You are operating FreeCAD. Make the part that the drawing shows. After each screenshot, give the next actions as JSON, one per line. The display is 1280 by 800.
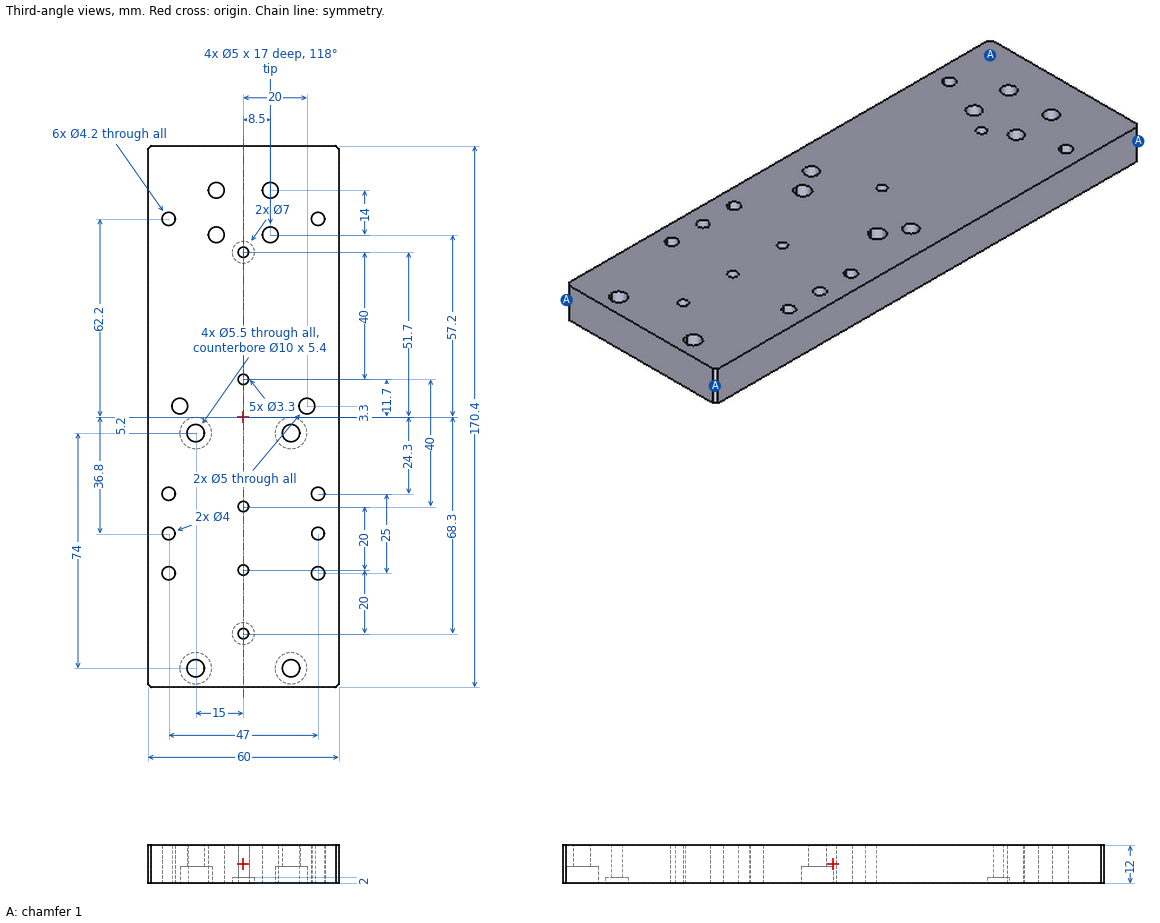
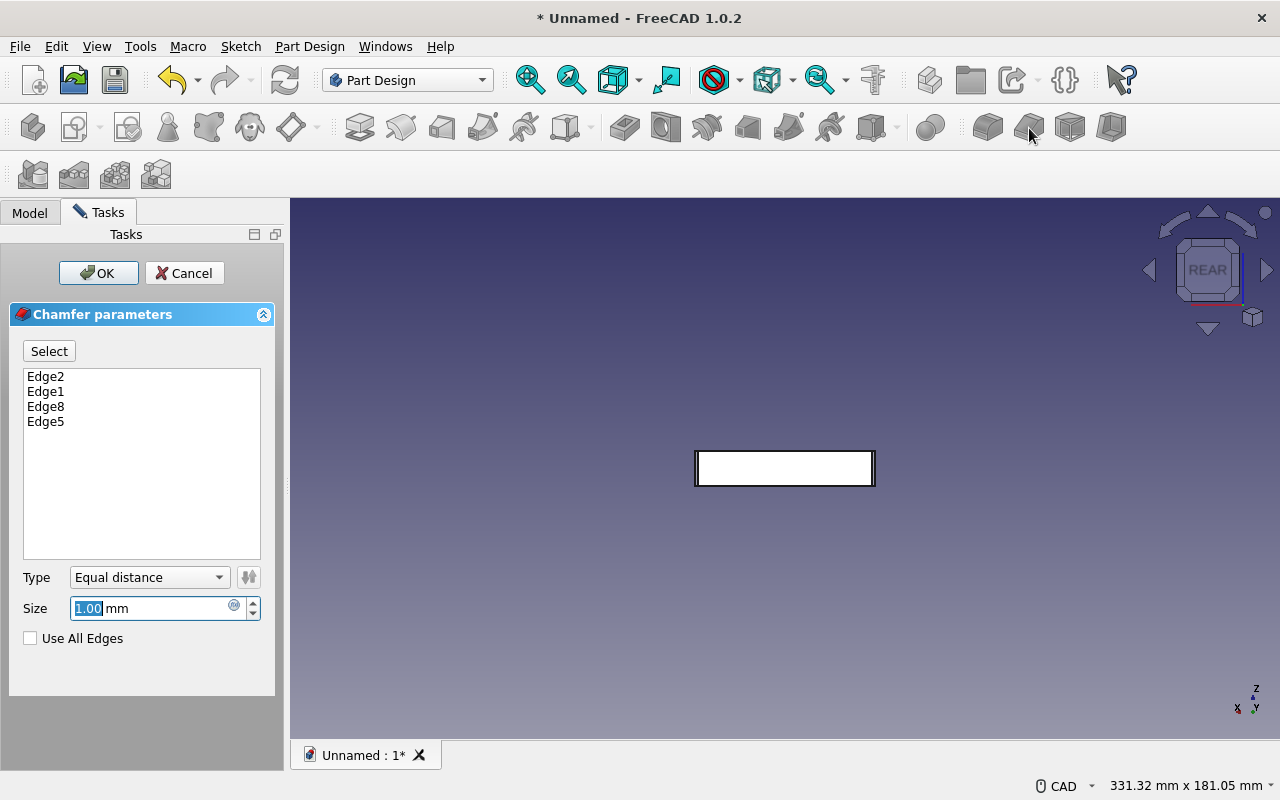
{"action": "type", "text": "1"}
{"action": "key", "text": "Tab"}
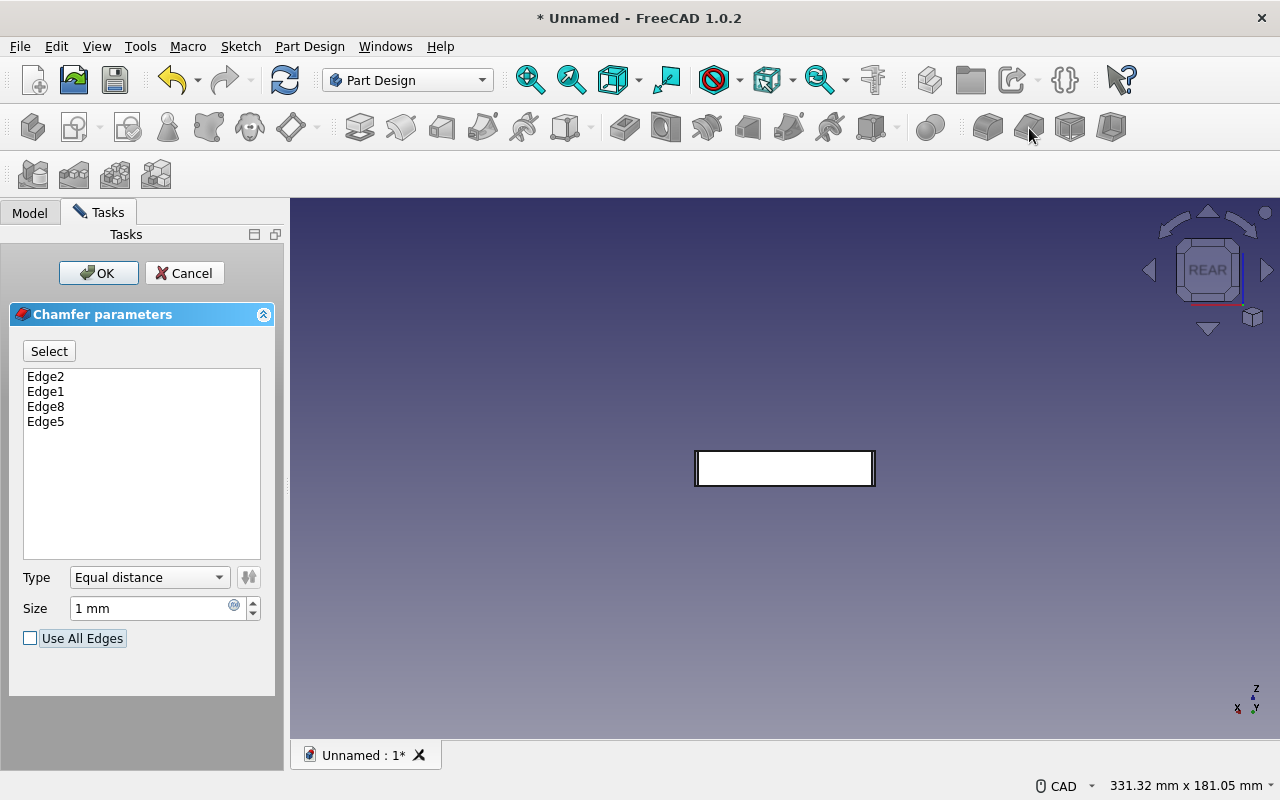
{"action": "left_click", "coordinate": [99, 273]}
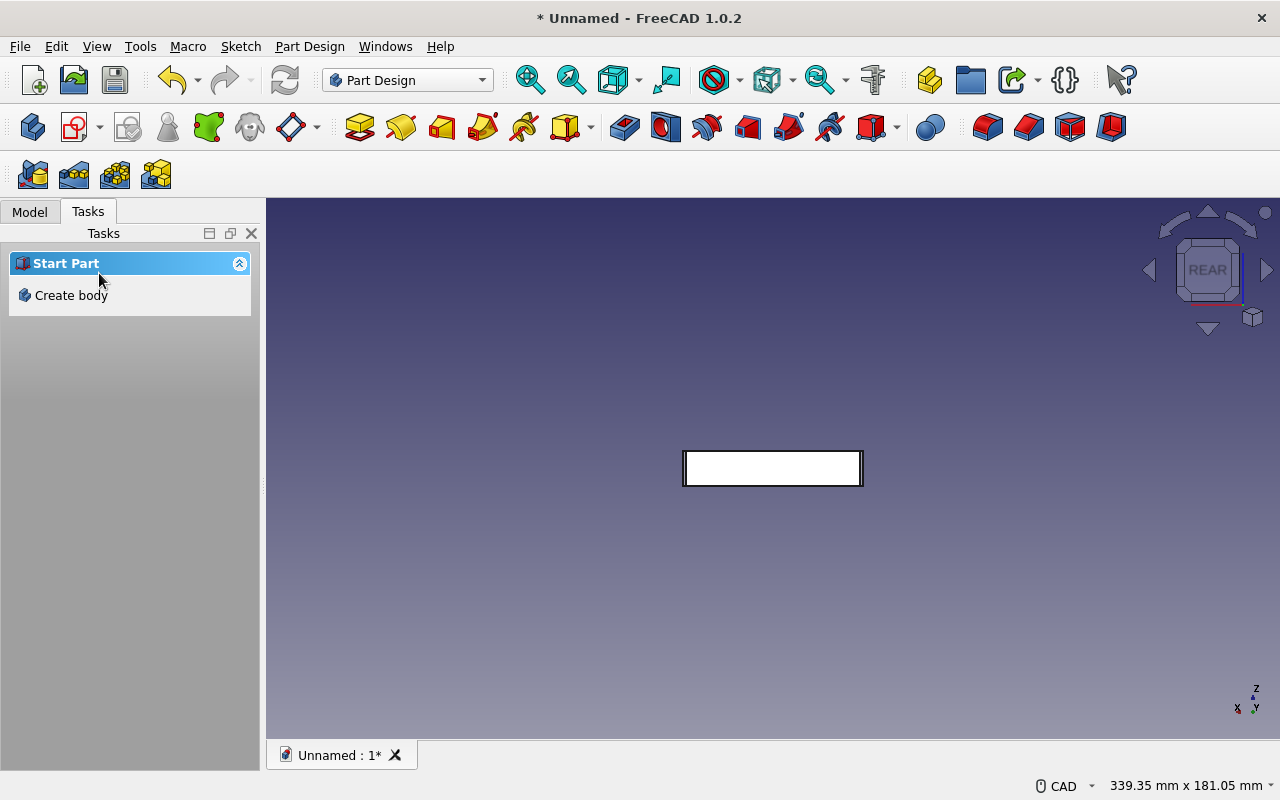
{"action": "left_click", "coordinate": [531, 80]}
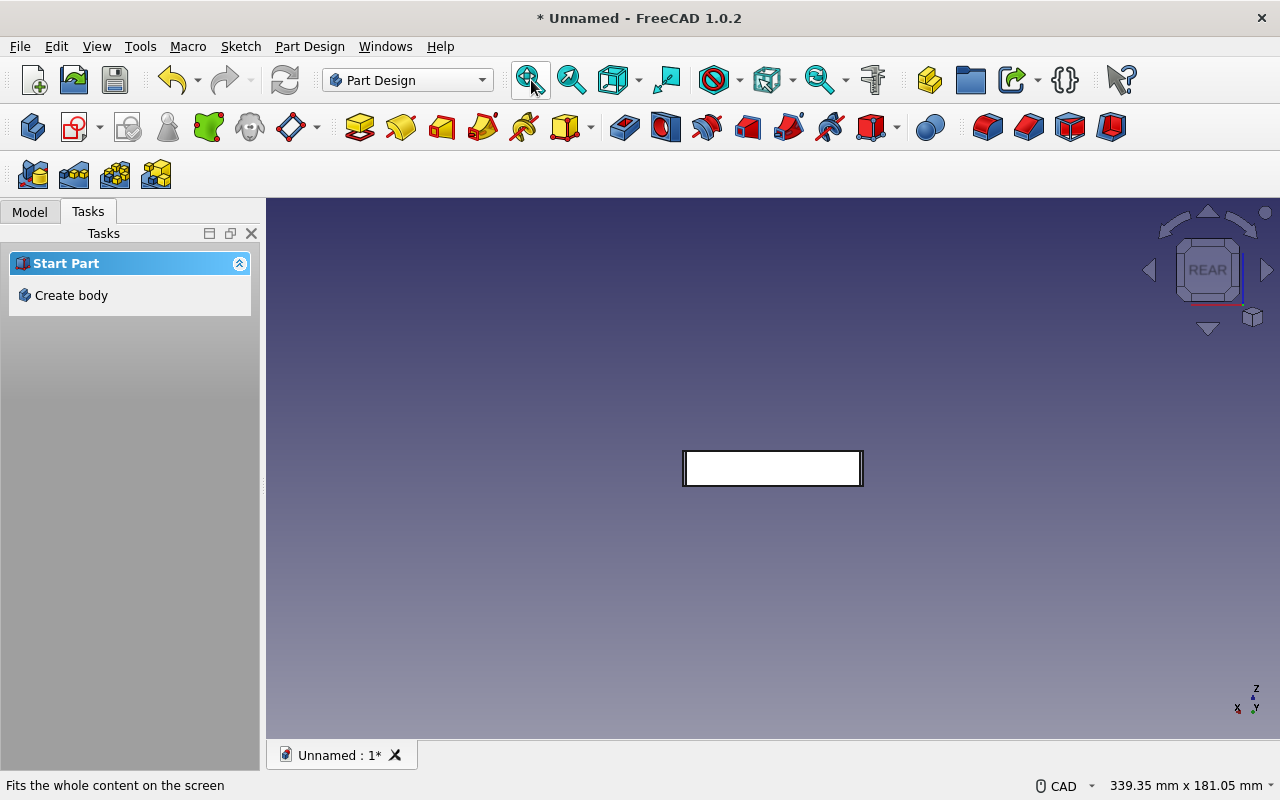
{"action": "key", "text": "5"}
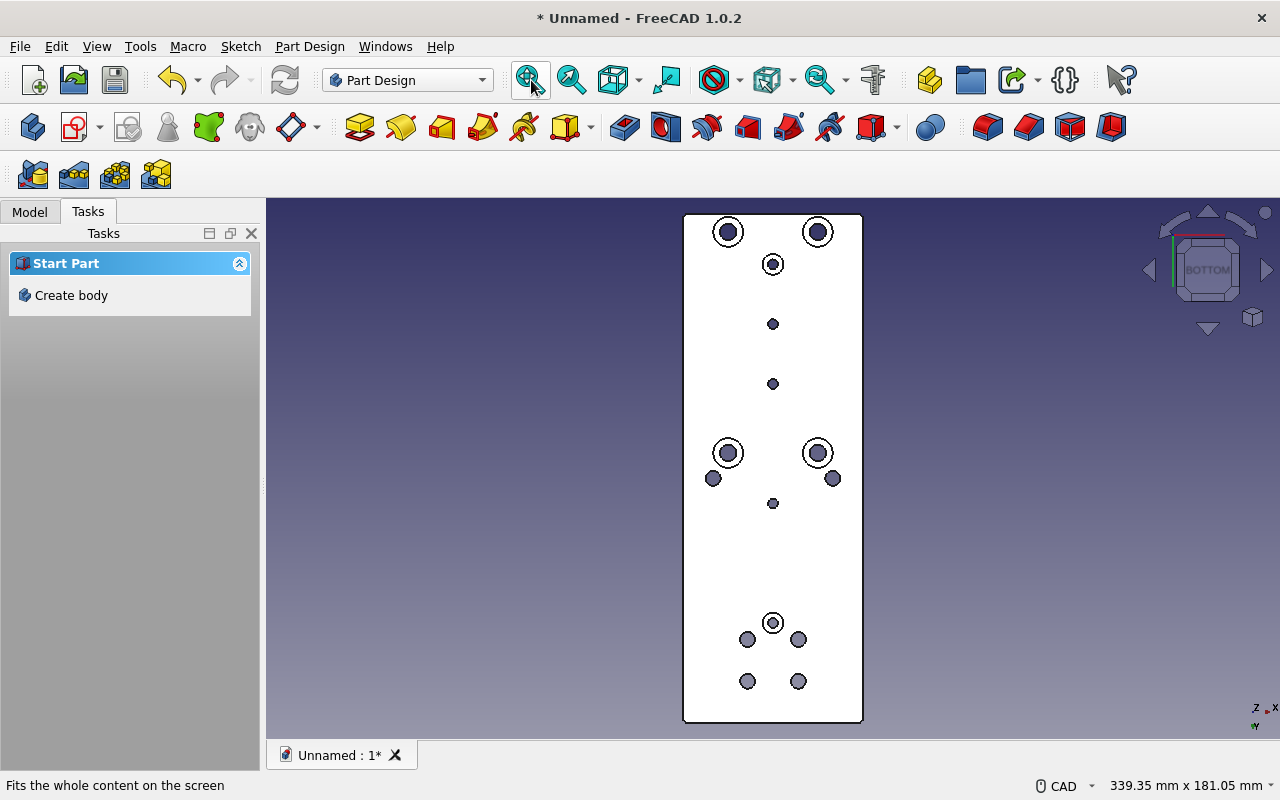
{"action": "left_click", "coordinate": [747, 540]}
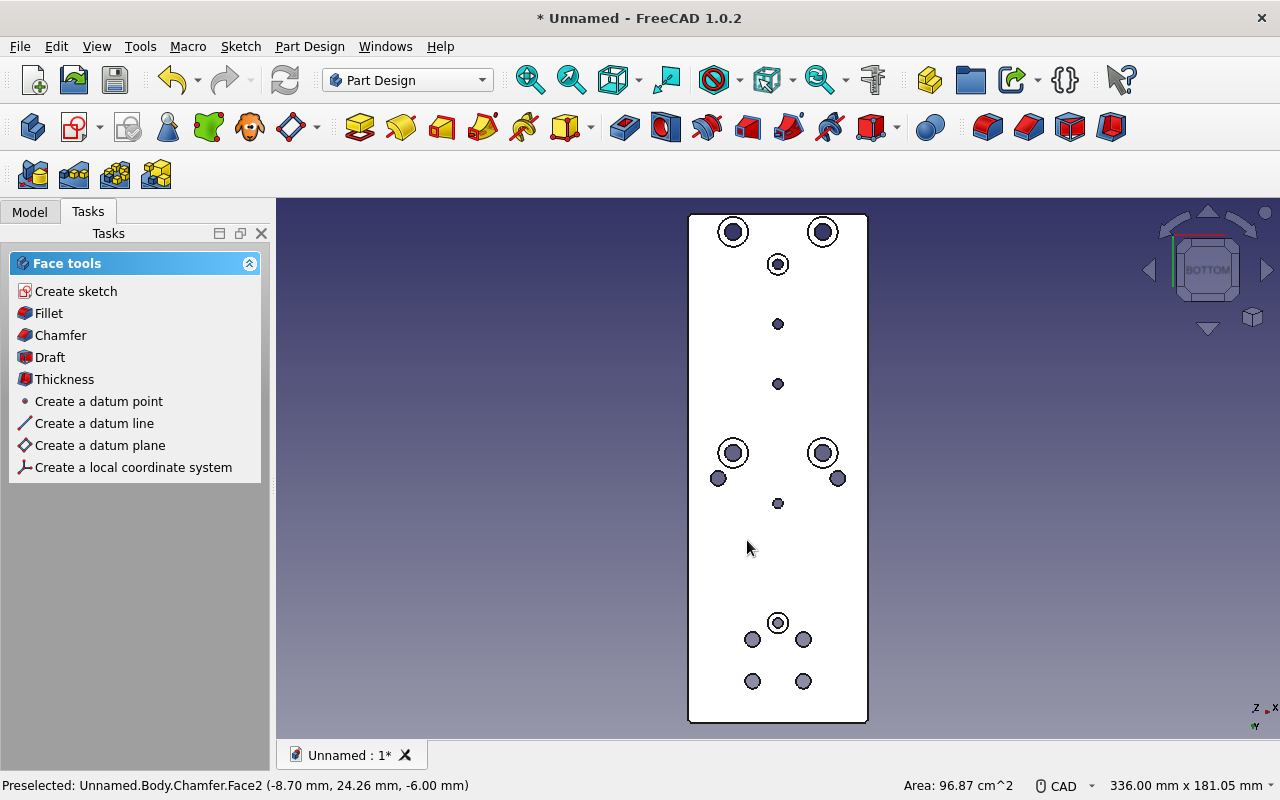
{"action": "left_click", "coordinate": [74, 128]}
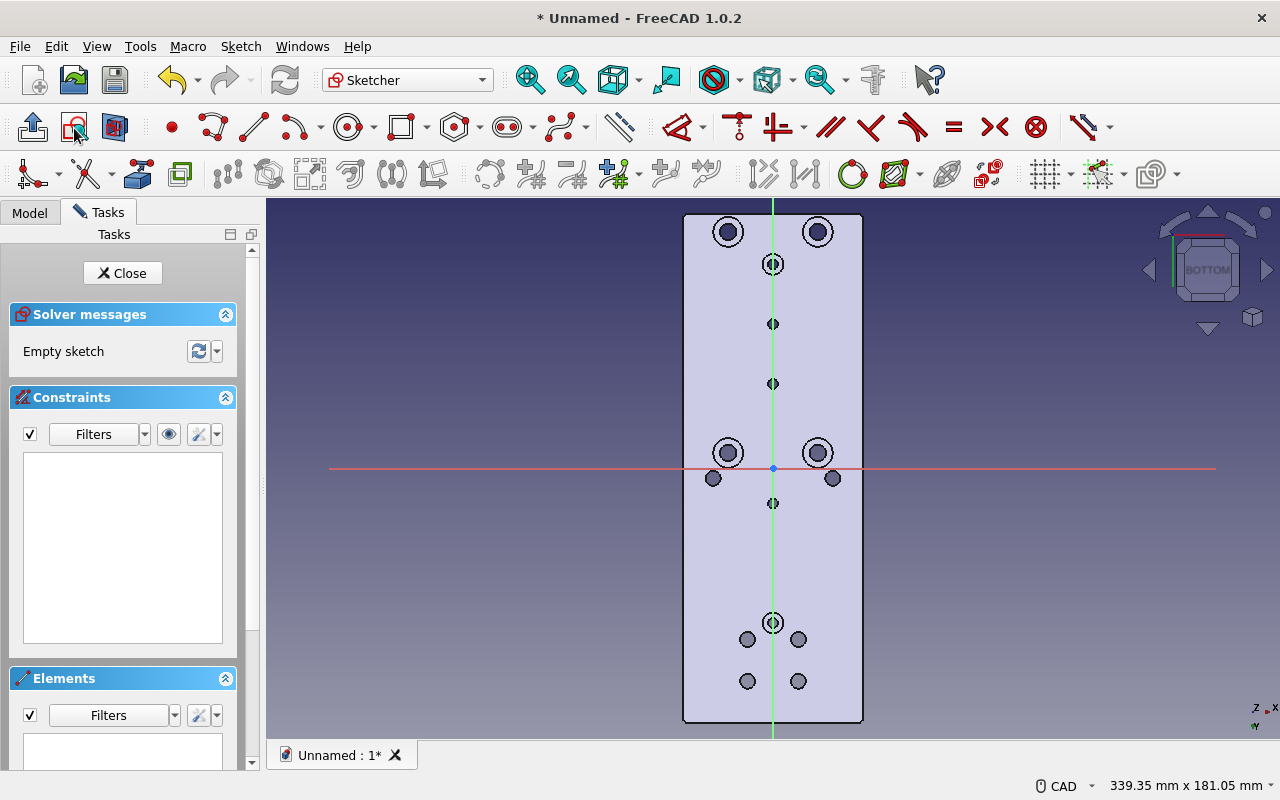
{"action": "scroll", "coordinate": [813, 377], "scroll_direction": "up", "scroll_amount": 5}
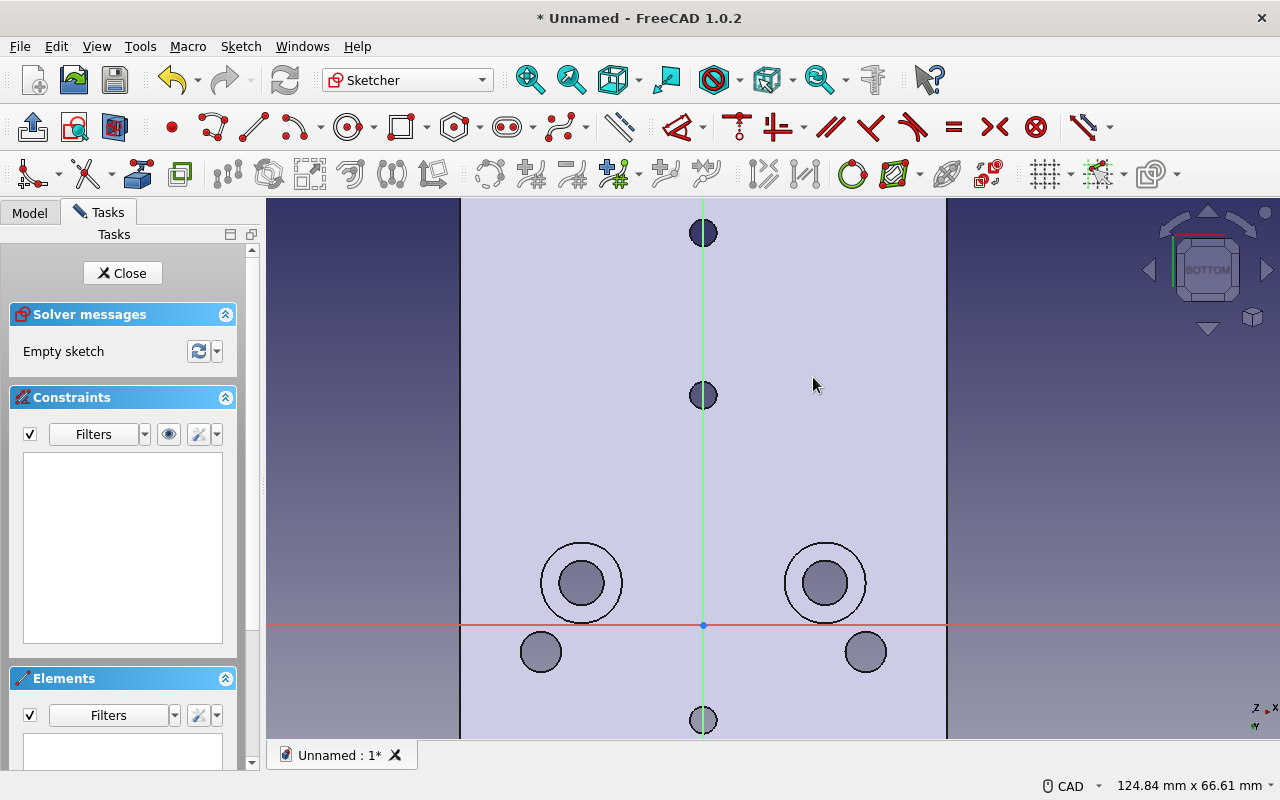
{"action": "left_click", "coordinate": [348, 128]}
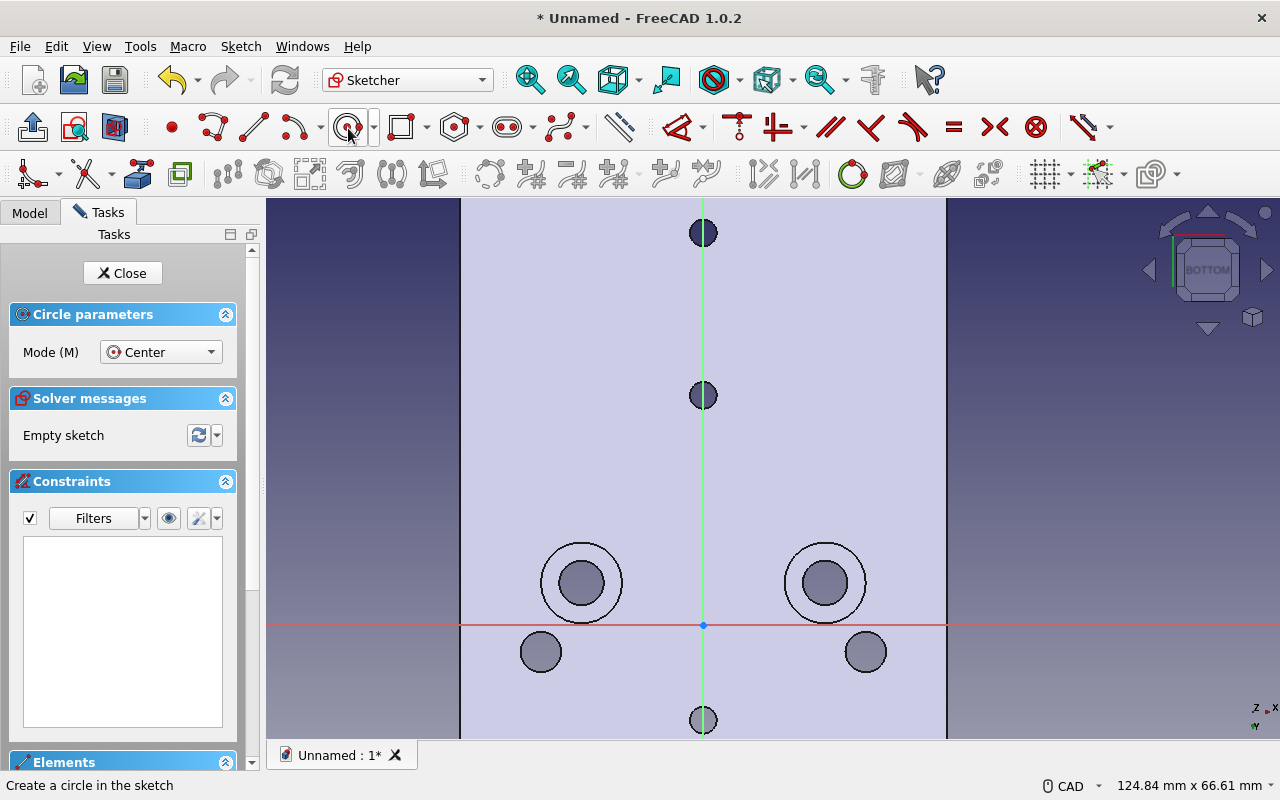
{"action": "scroll", "coordinate": [512, 326], "scroll_direction": "up", "scroll_amount": 2}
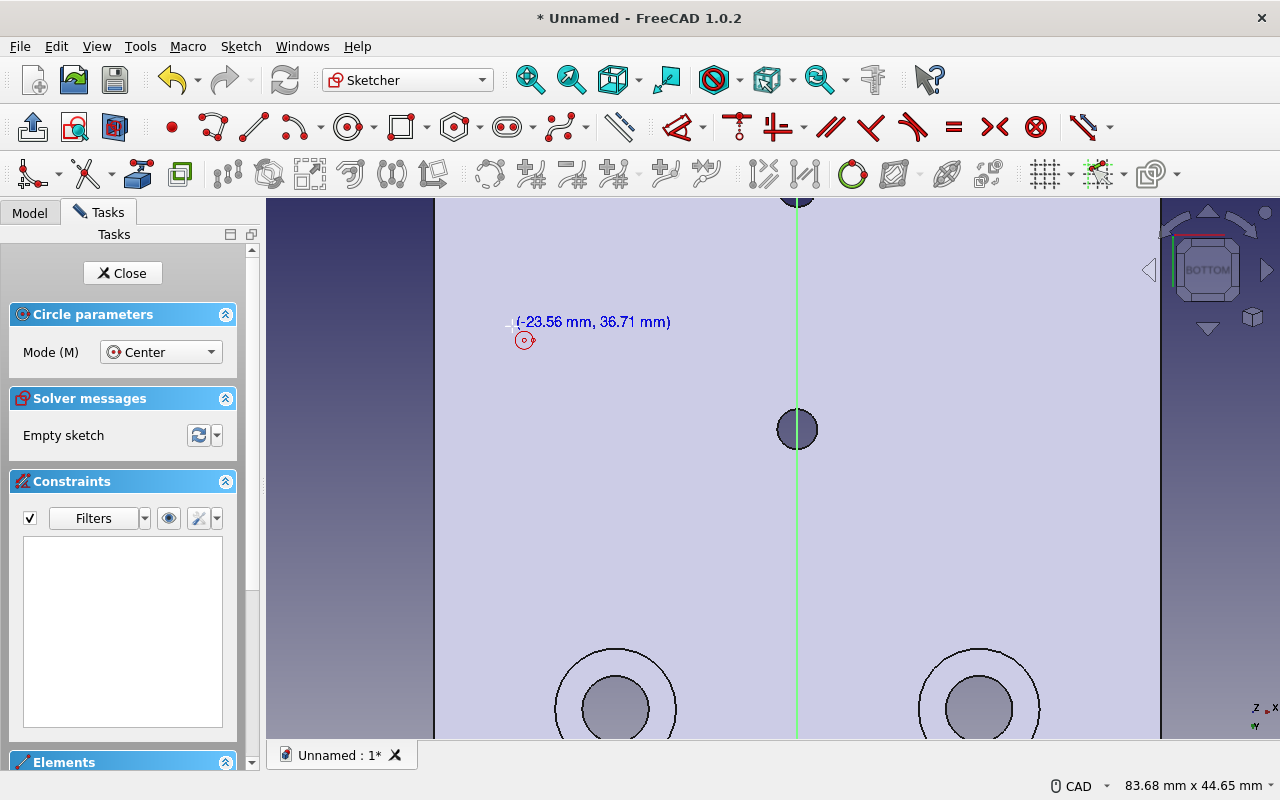
{"action": "left_click", "coordinate": [513, 326]}
{"action": "left_click", "coordinate": [530, 309]}